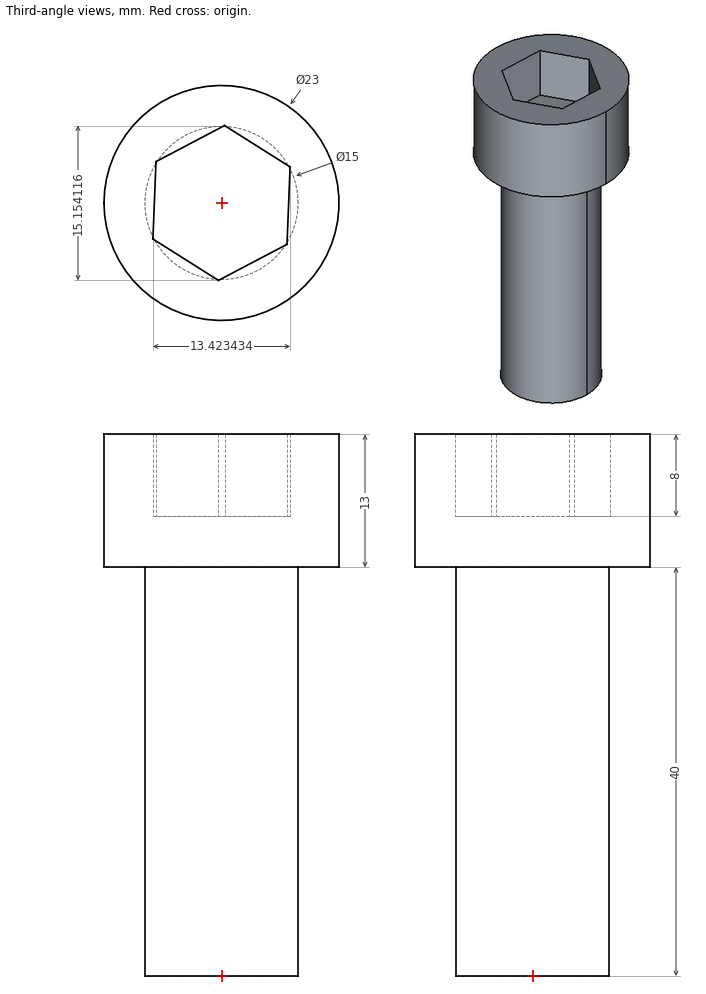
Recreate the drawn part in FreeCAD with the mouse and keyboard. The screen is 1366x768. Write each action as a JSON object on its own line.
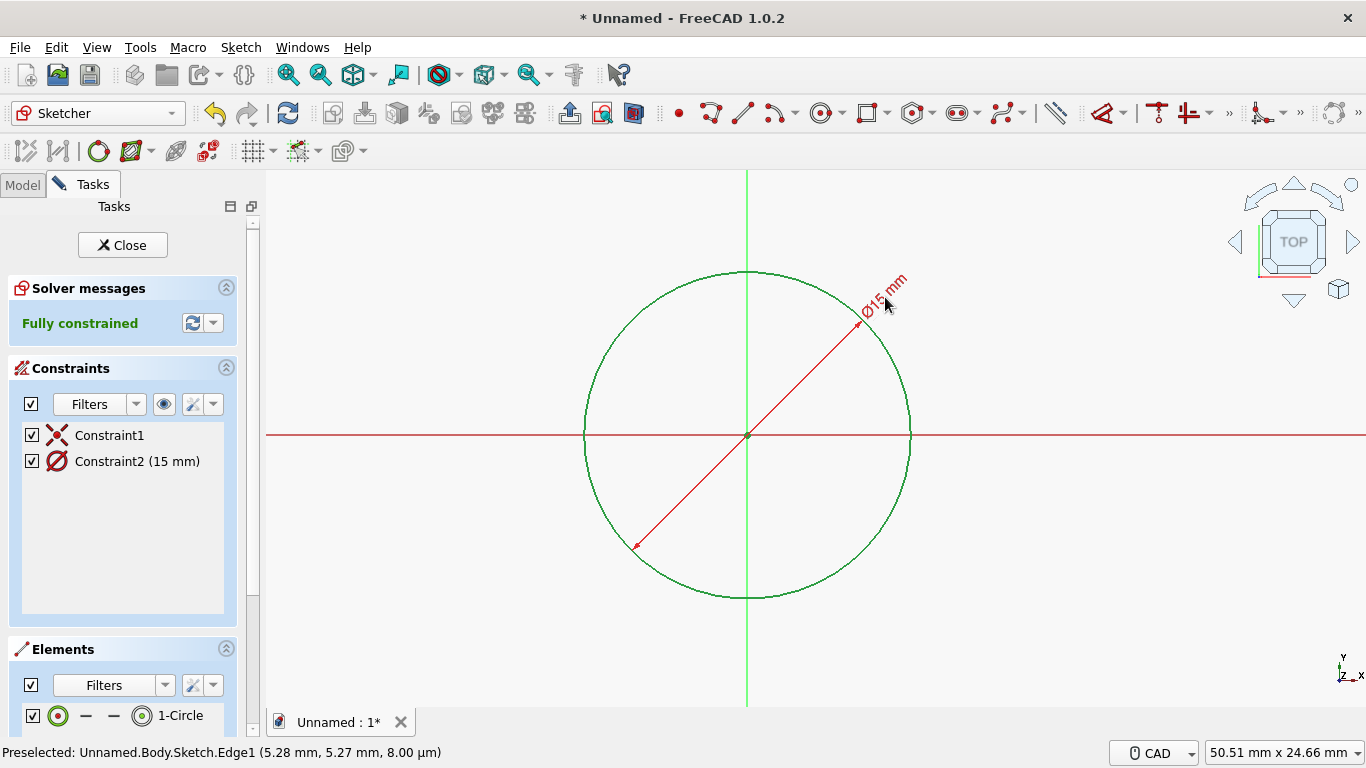
{"action": "left_click", "coordinate": [123, 245]}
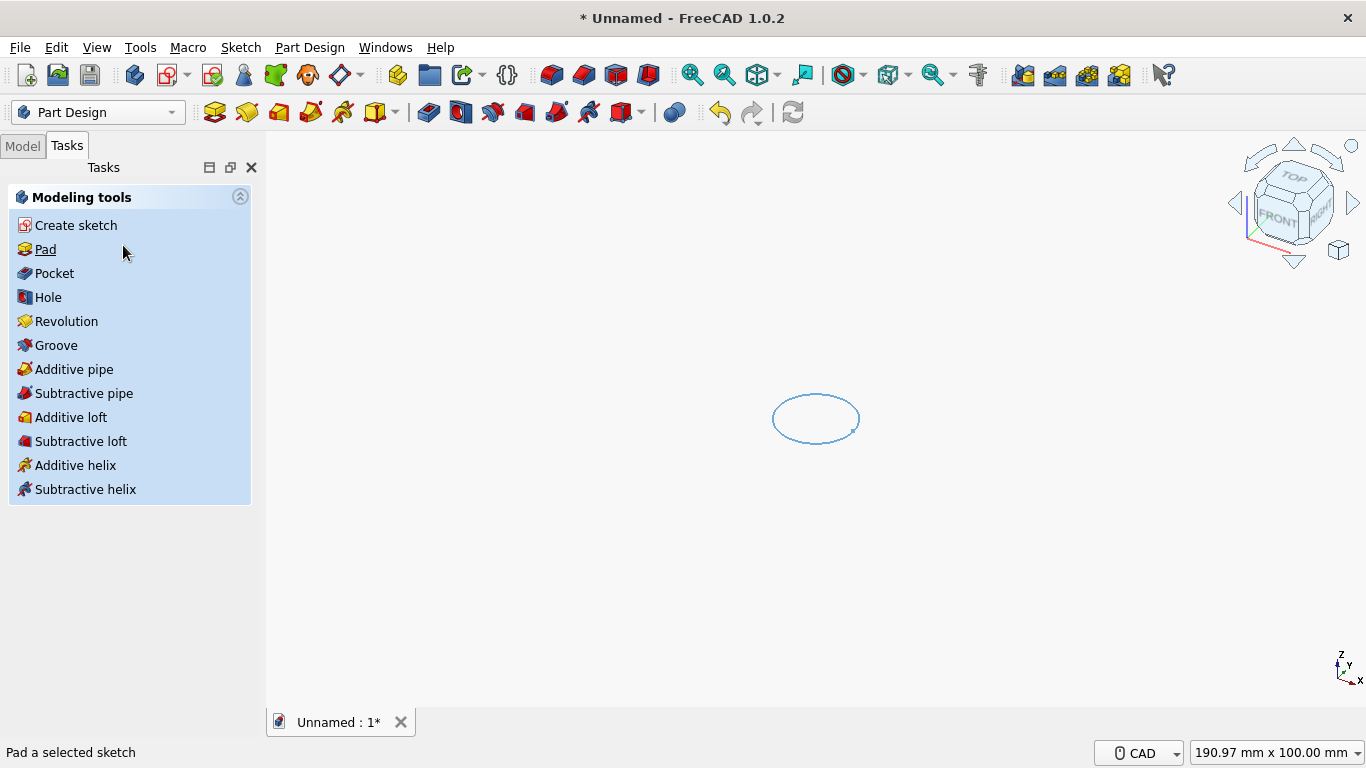
{"action": "left_click", "coordinate": [216, 112]}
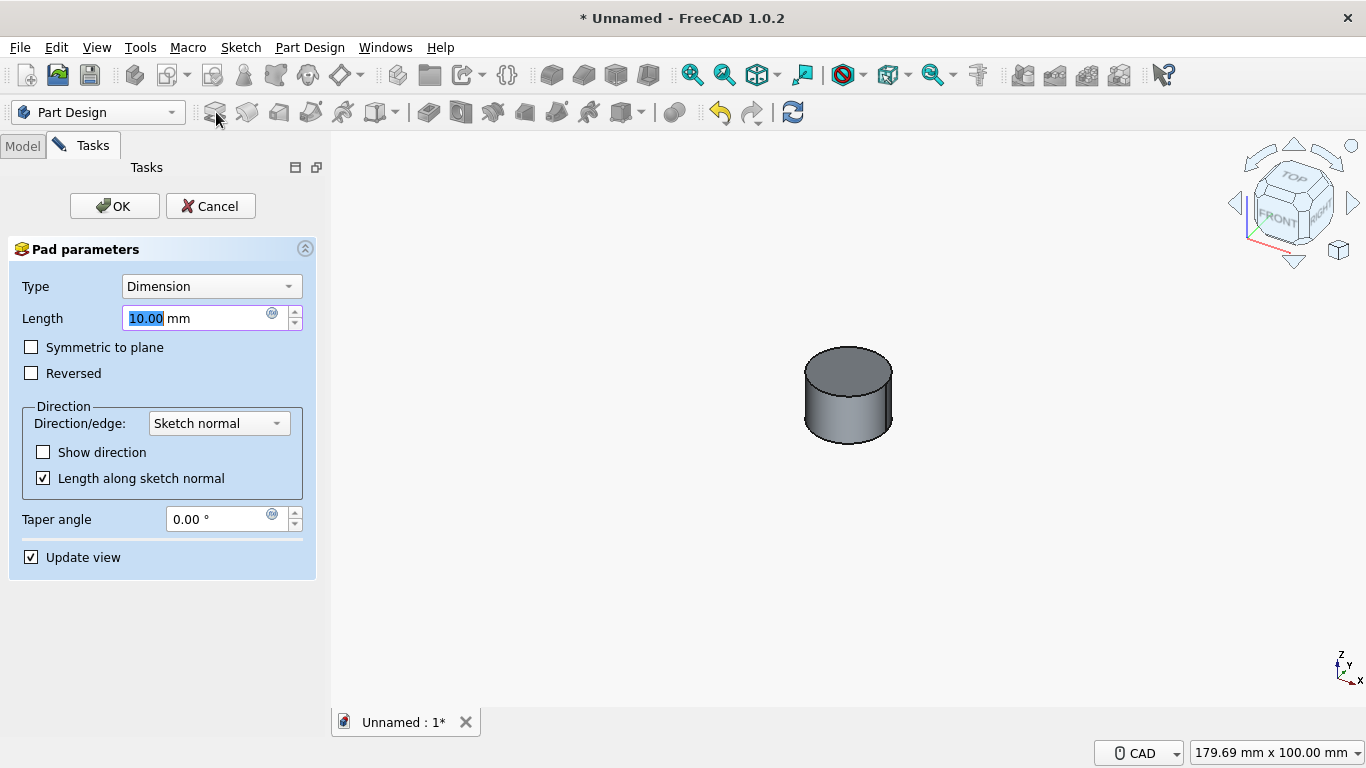
{"action": "type", "text": "40"}
{"action": "key", "text": "Tab"}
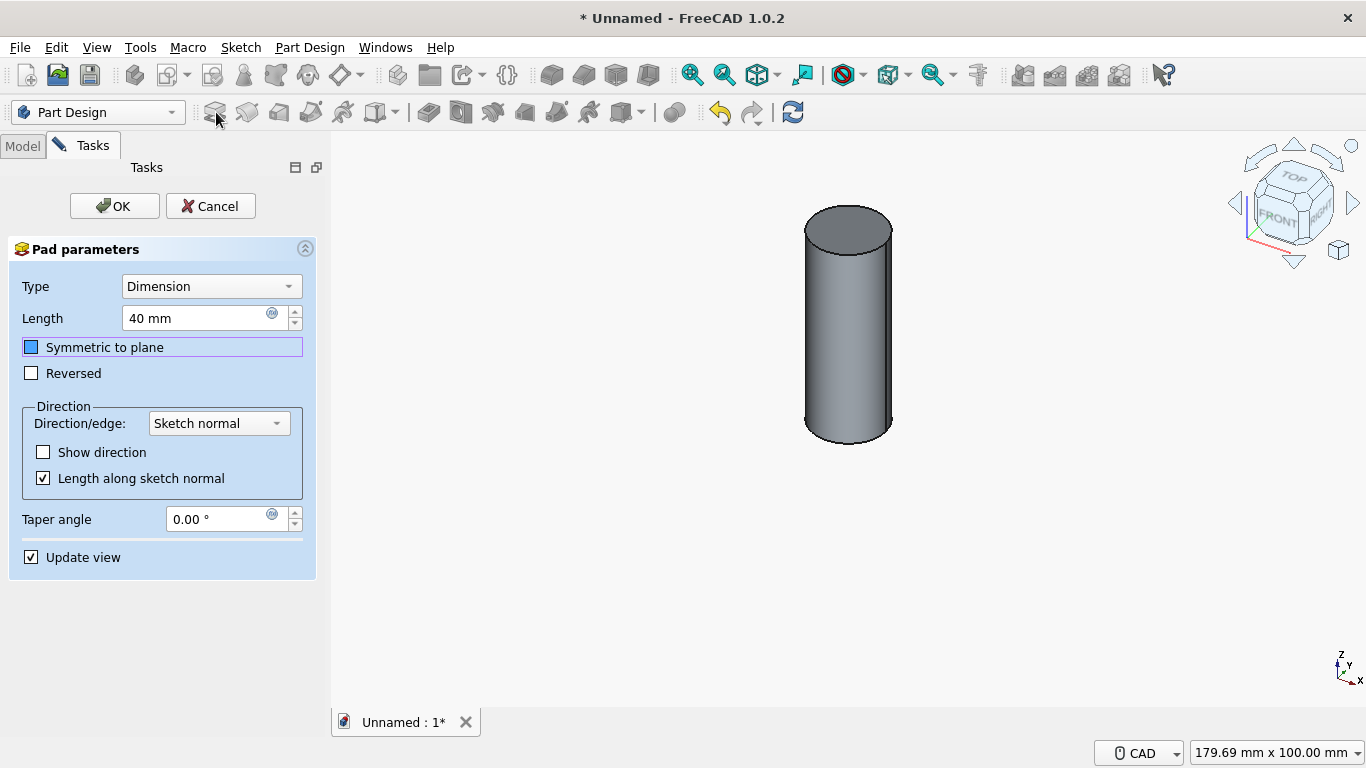
{"action": "left_click", "coordinate": [115, 206]}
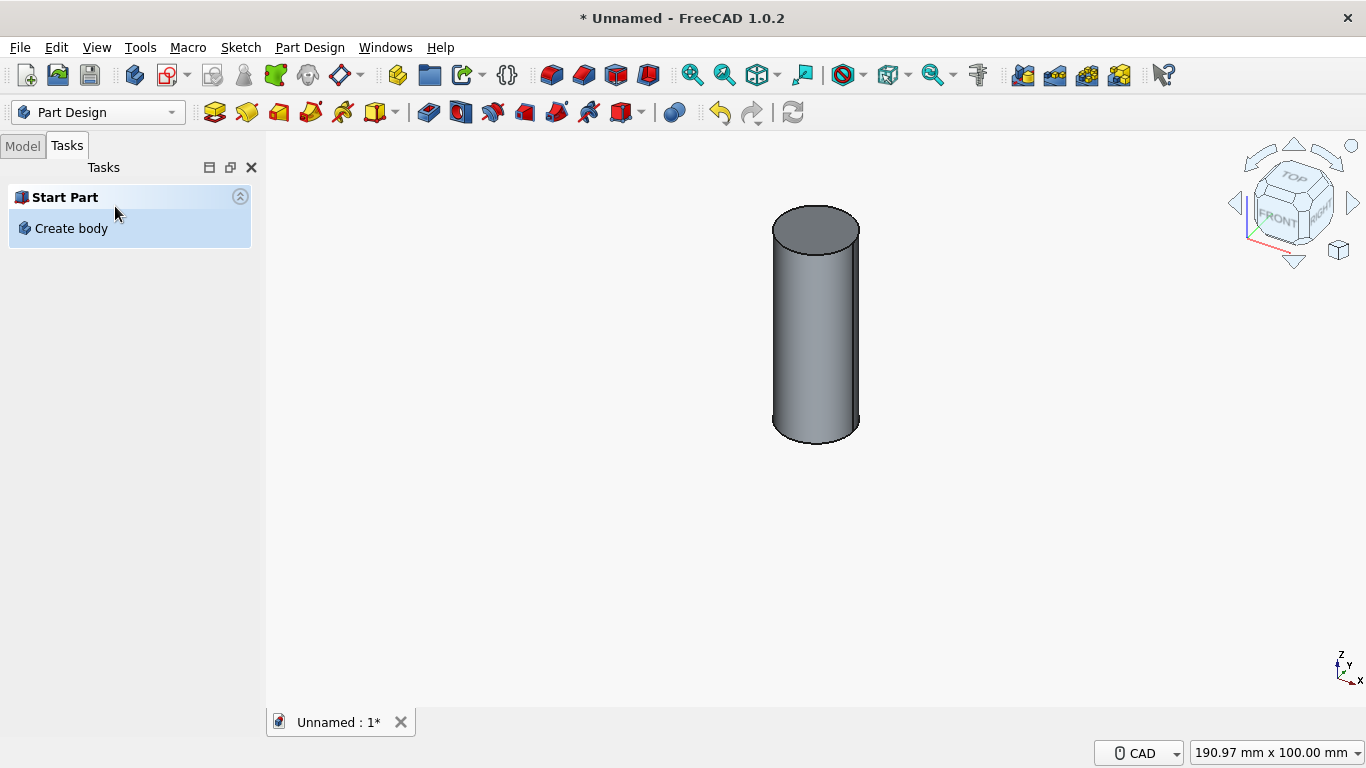
{"action": "left_click", "coordinate": [694, 76]}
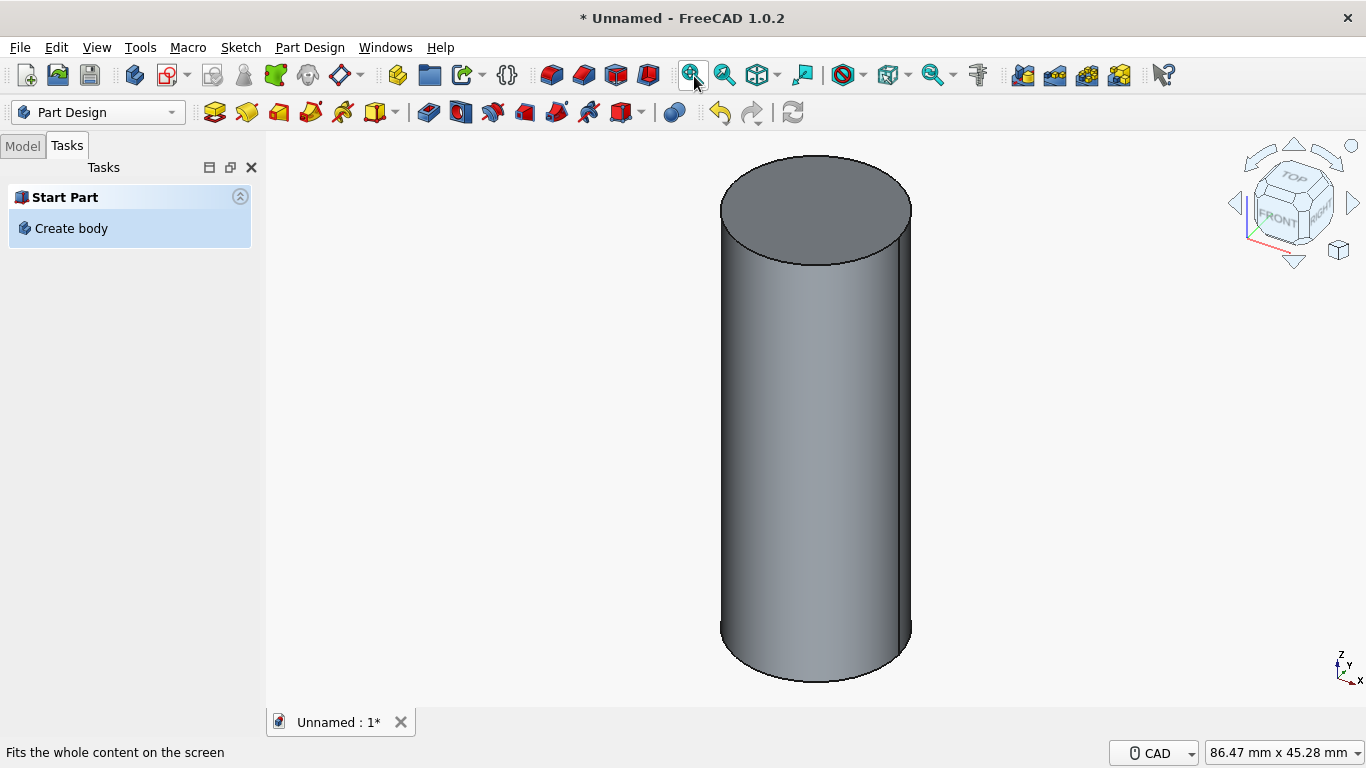
{"action": "left_click", "coordinate": [816, 210]}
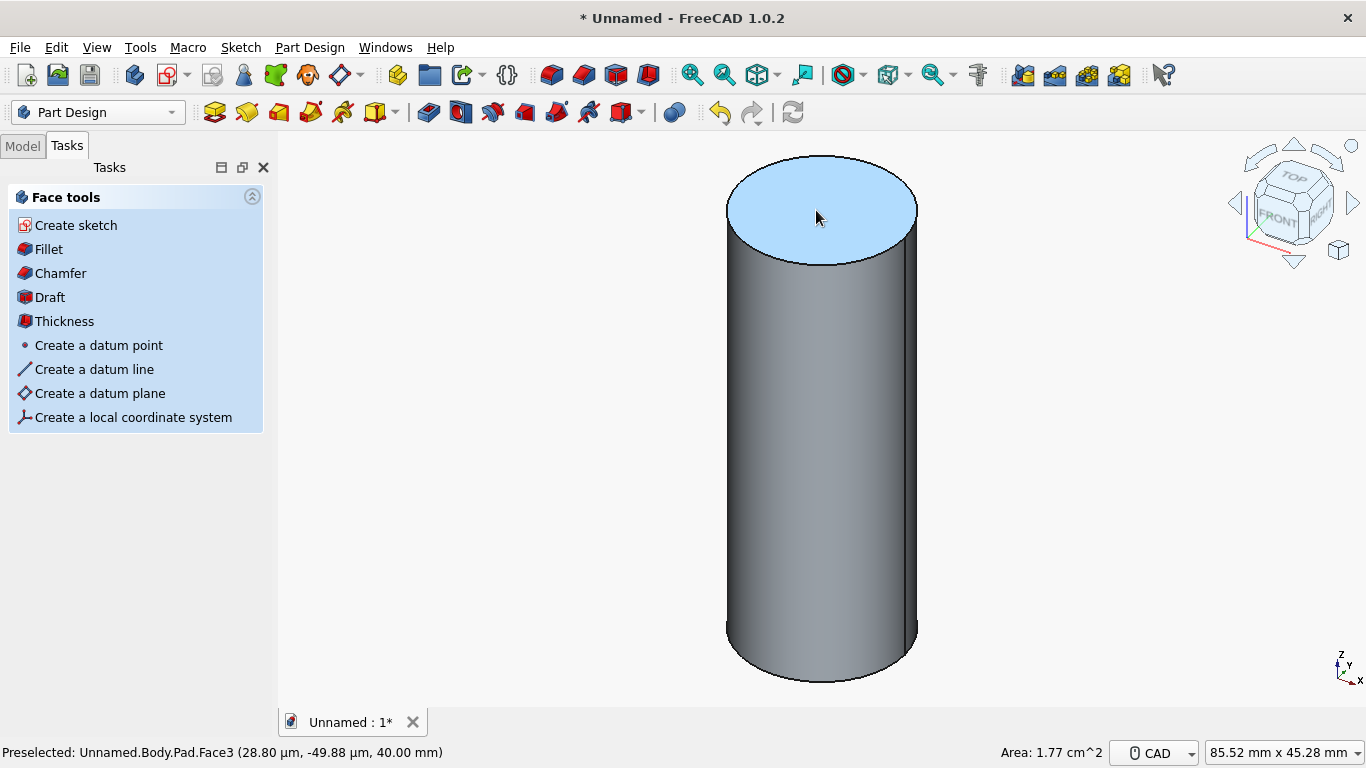
{"action": "left_click", "coordinate": [168, 76]}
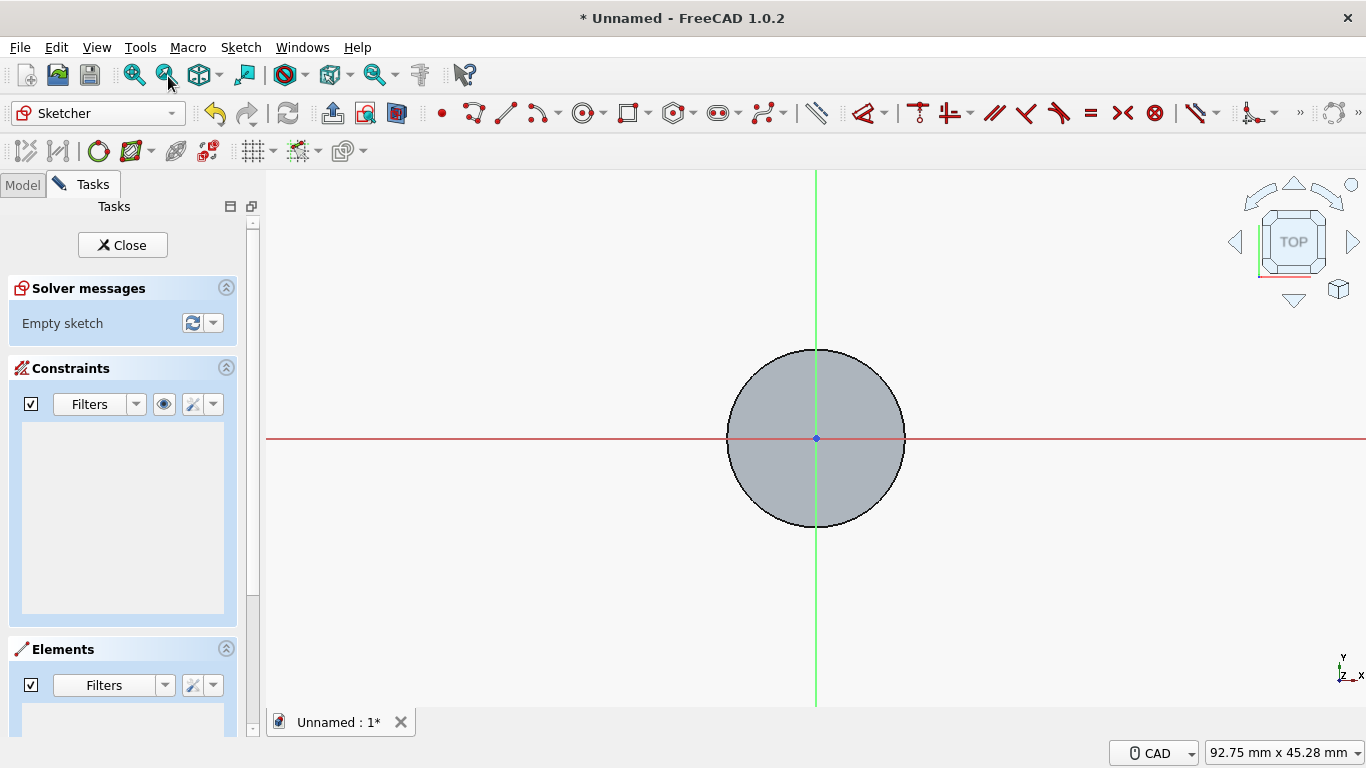
{"action": "left_click", "coordinate": [584, 114]}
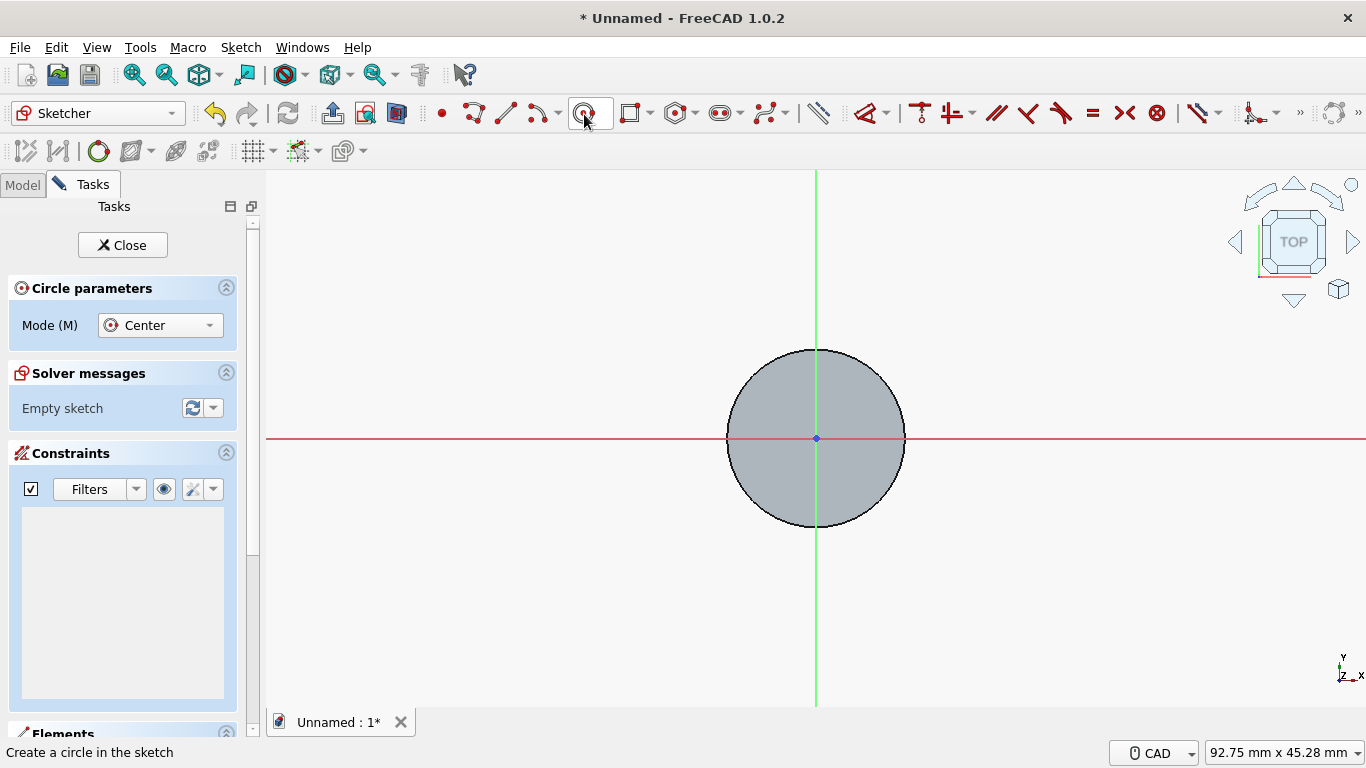
{"action": "left_click", "coordinate": [816, 438]}
{"action": "left_click", "coordinate": [912, 342]}
{"action": "key", "text": "Escape"}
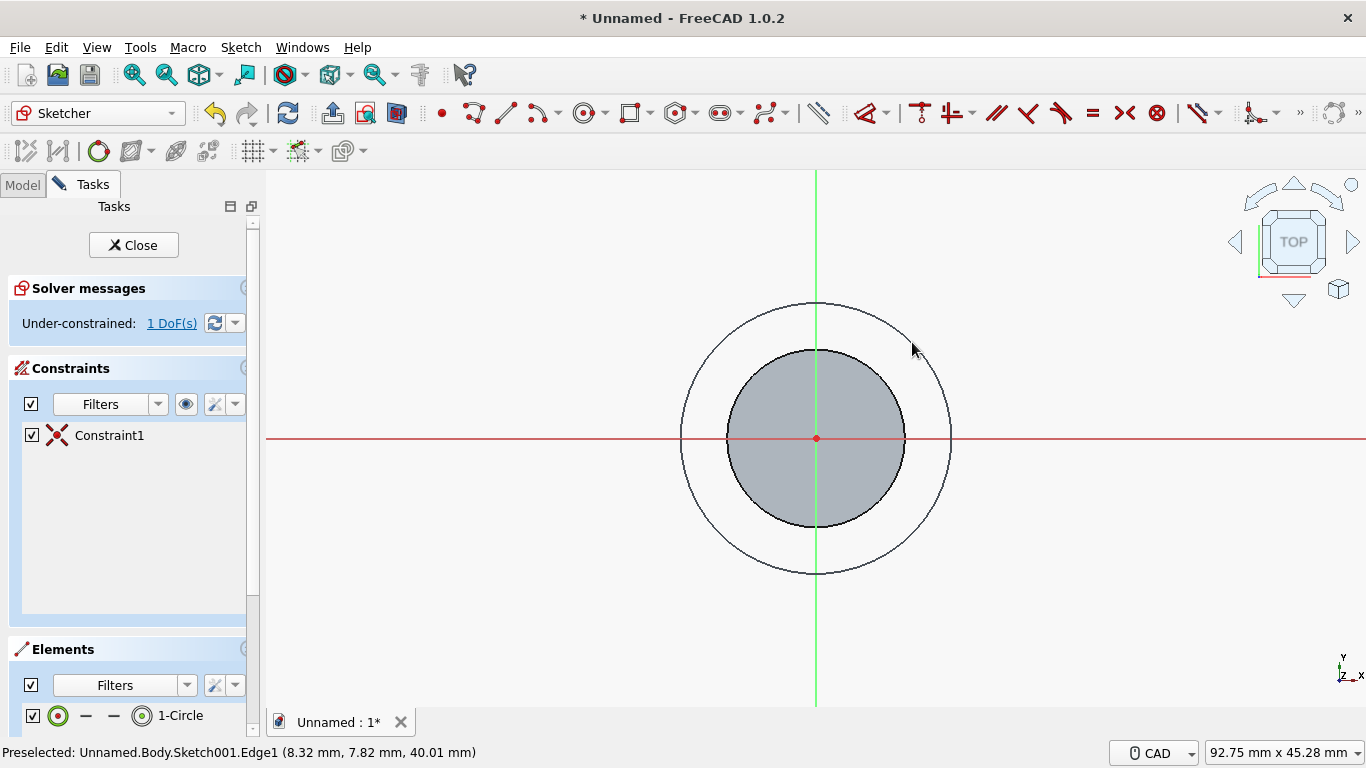
{"action": "left_click", "coordinate": [866, 114]}